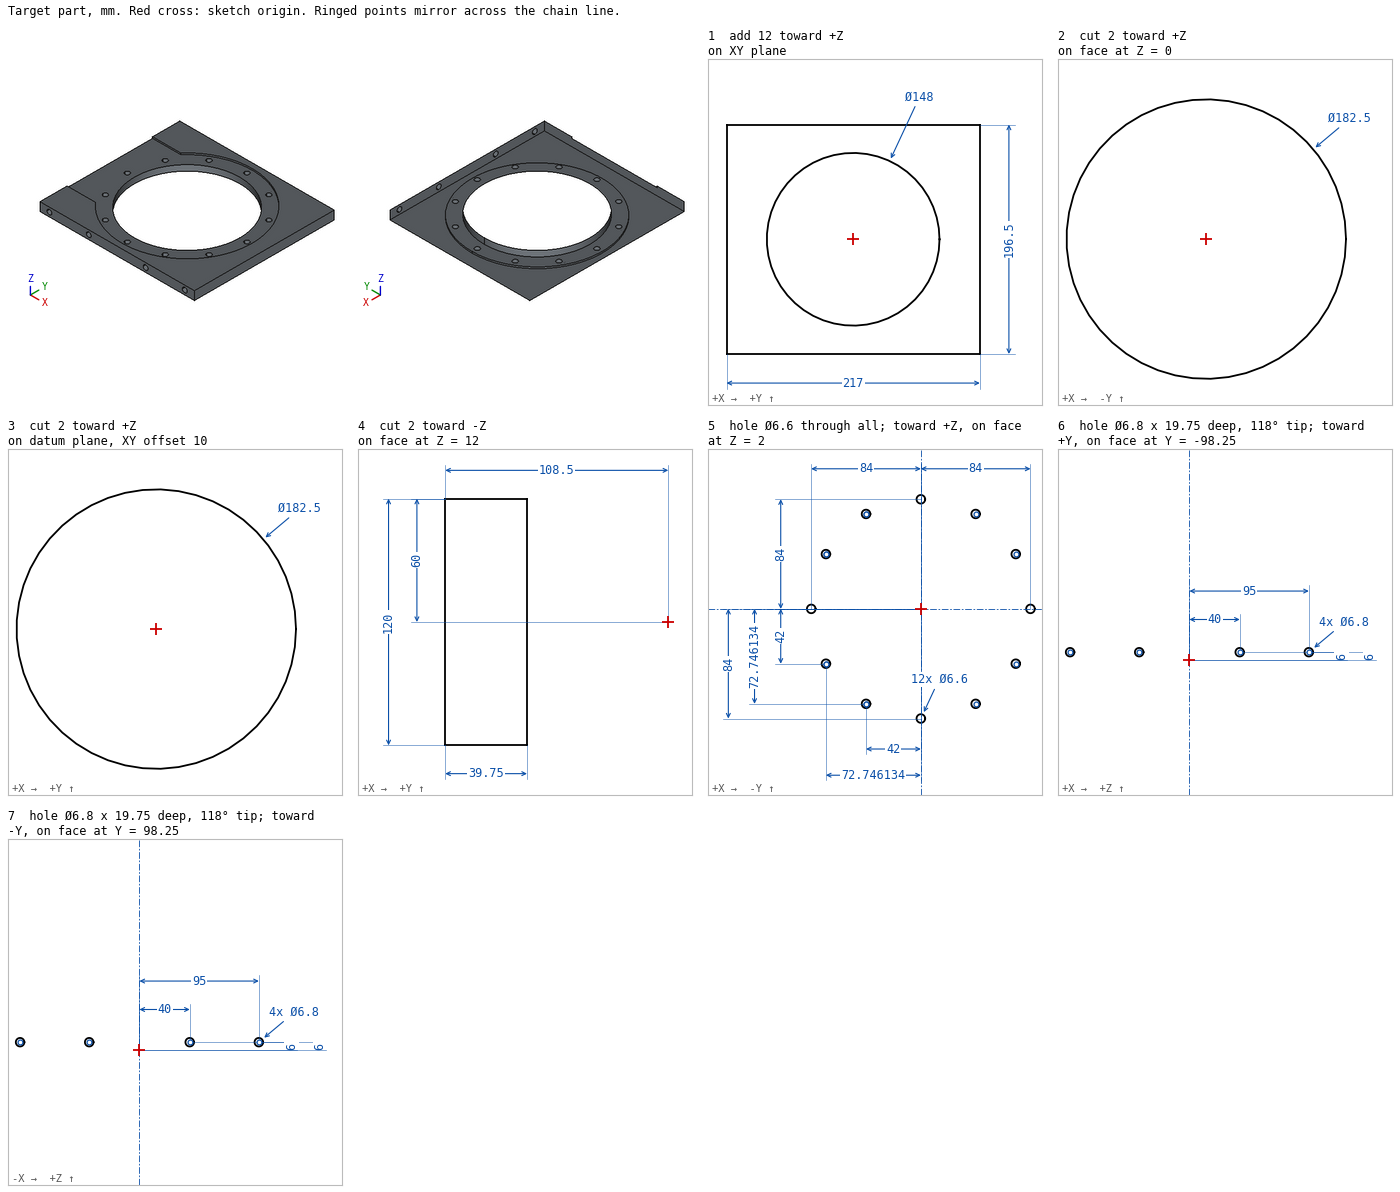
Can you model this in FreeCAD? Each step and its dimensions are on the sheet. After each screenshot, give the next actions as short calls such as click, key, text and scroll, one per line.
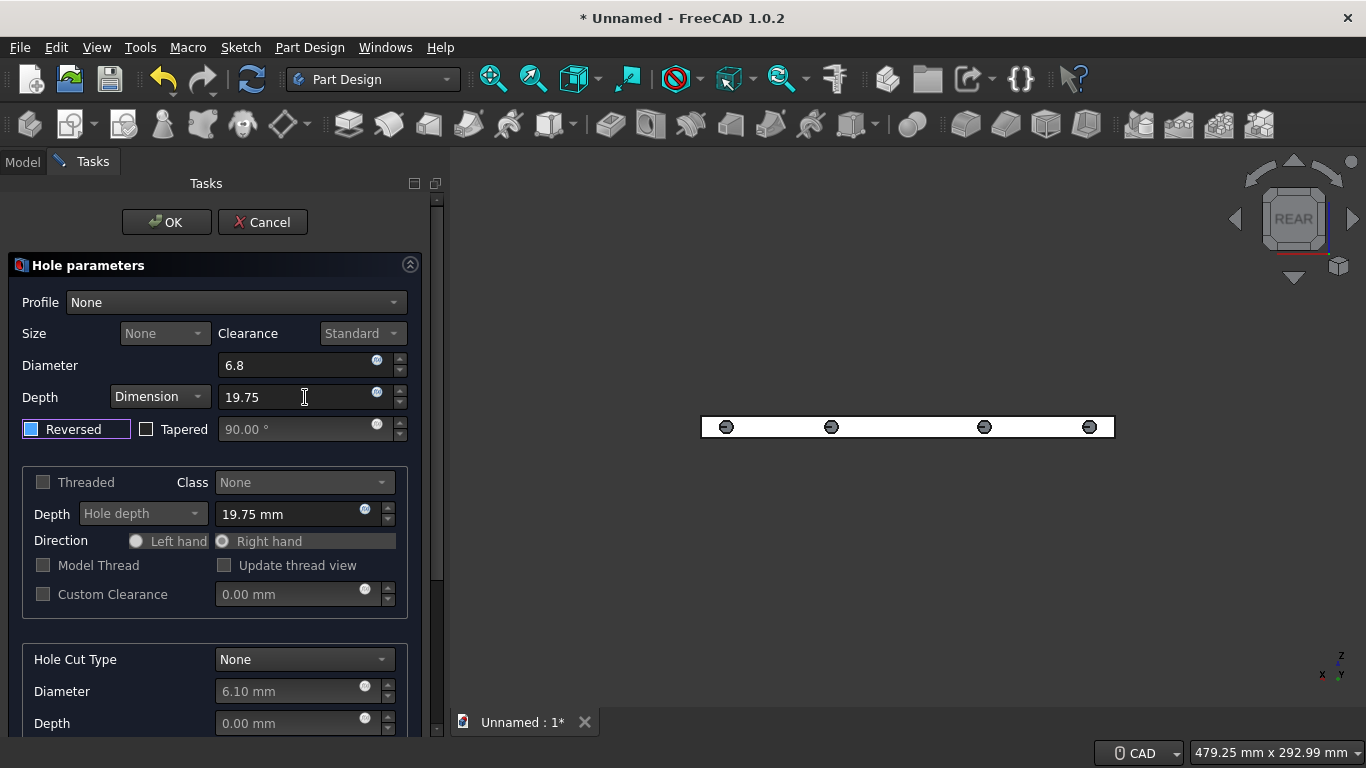
click(167, 222)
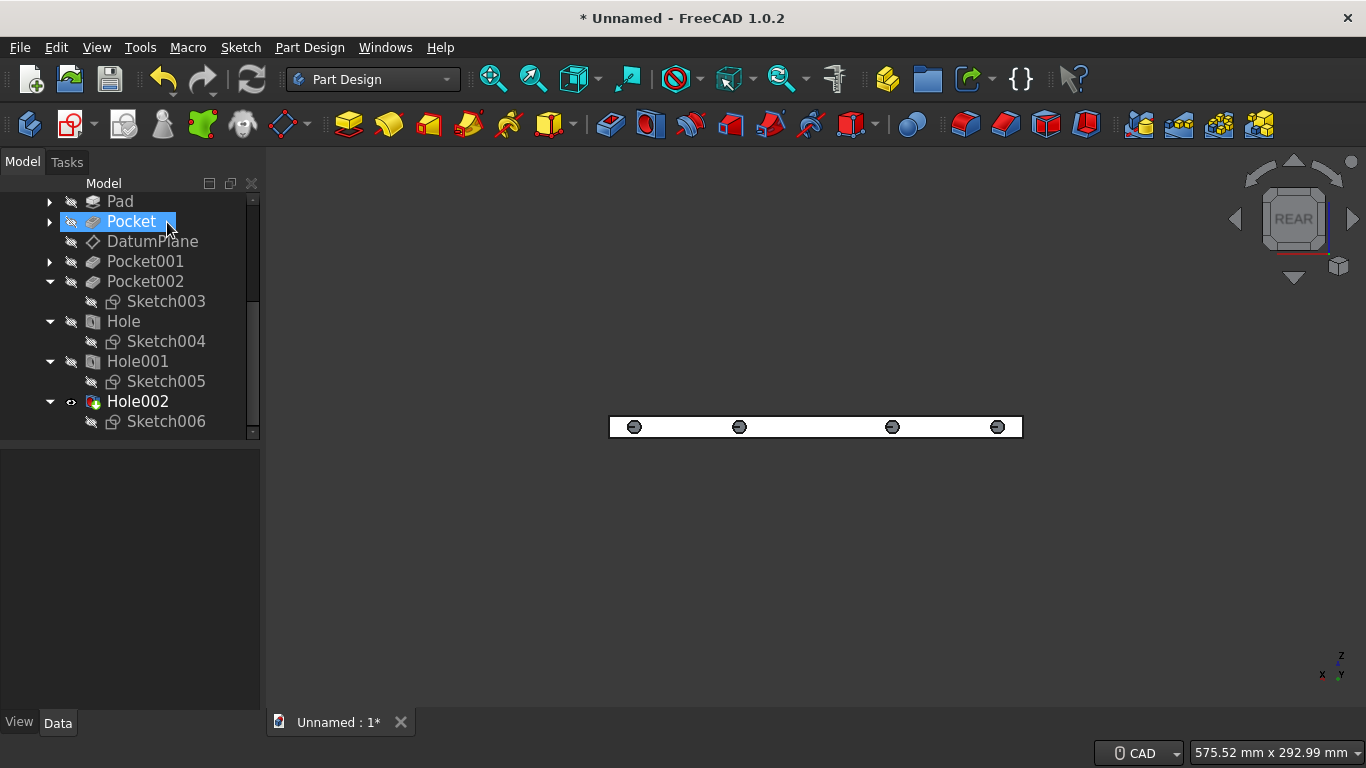
key(0)